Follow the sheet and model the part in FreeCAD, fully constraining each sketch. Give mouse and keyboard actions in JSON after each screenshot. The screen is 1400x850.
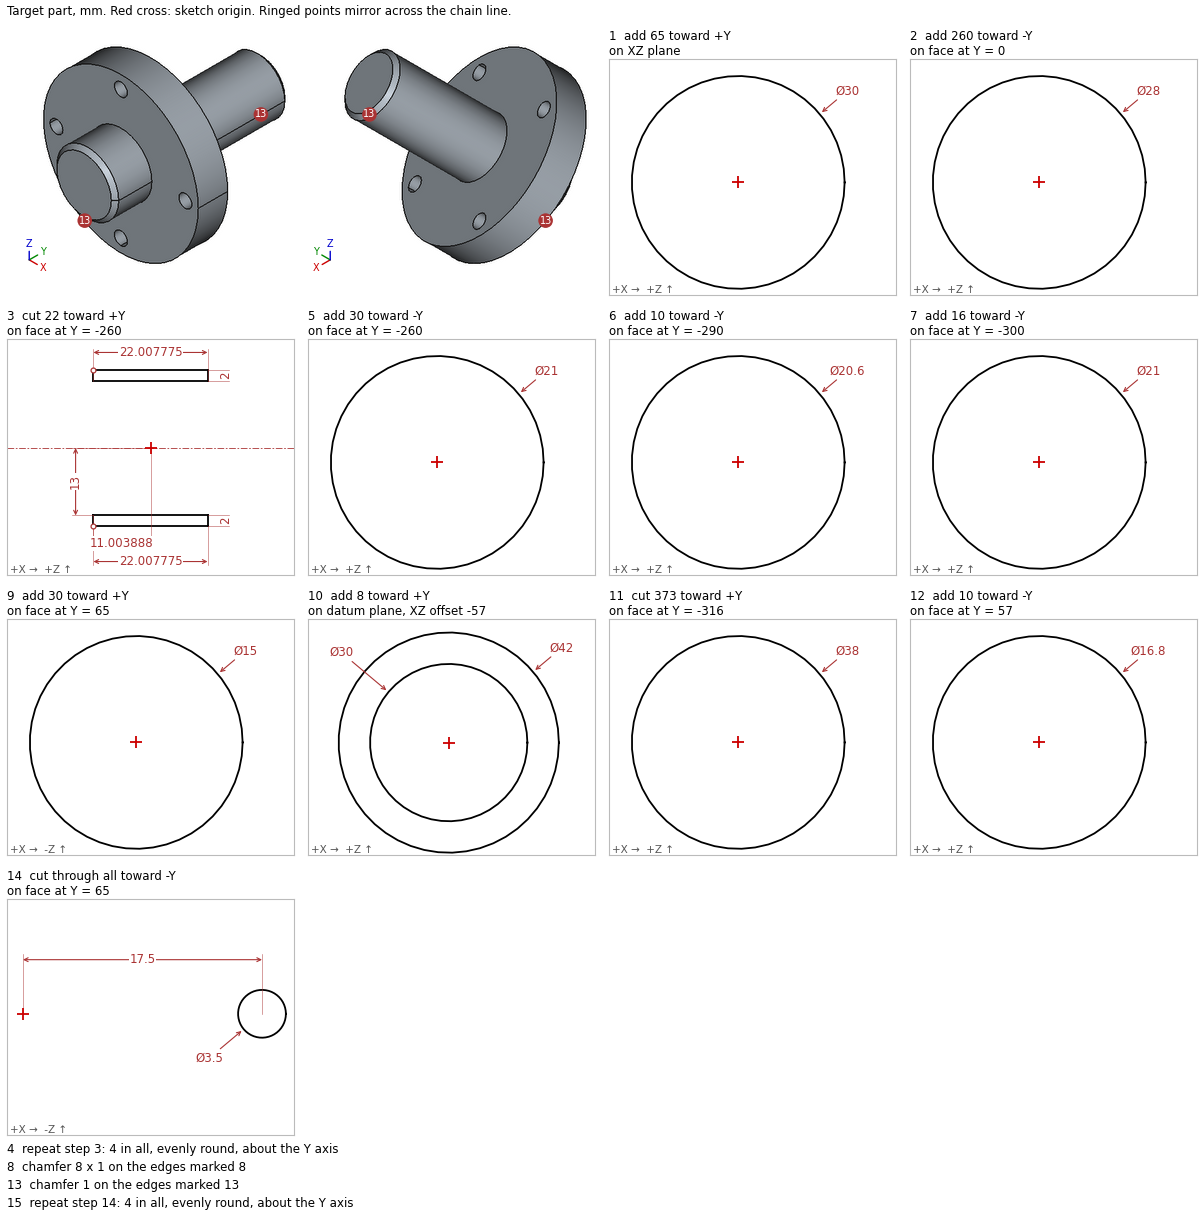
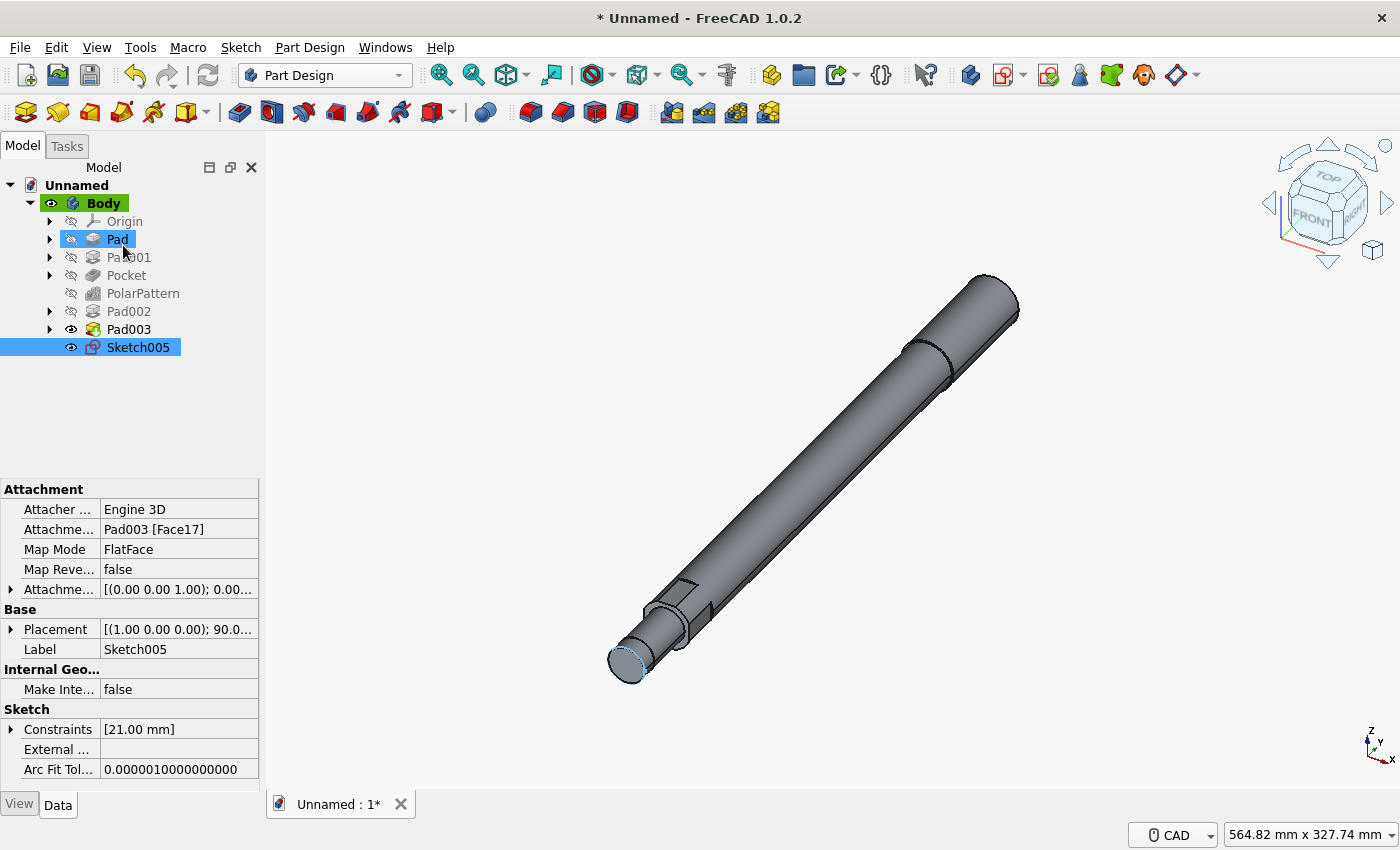
{"action": "left_click", "coordinate": [26, 112]}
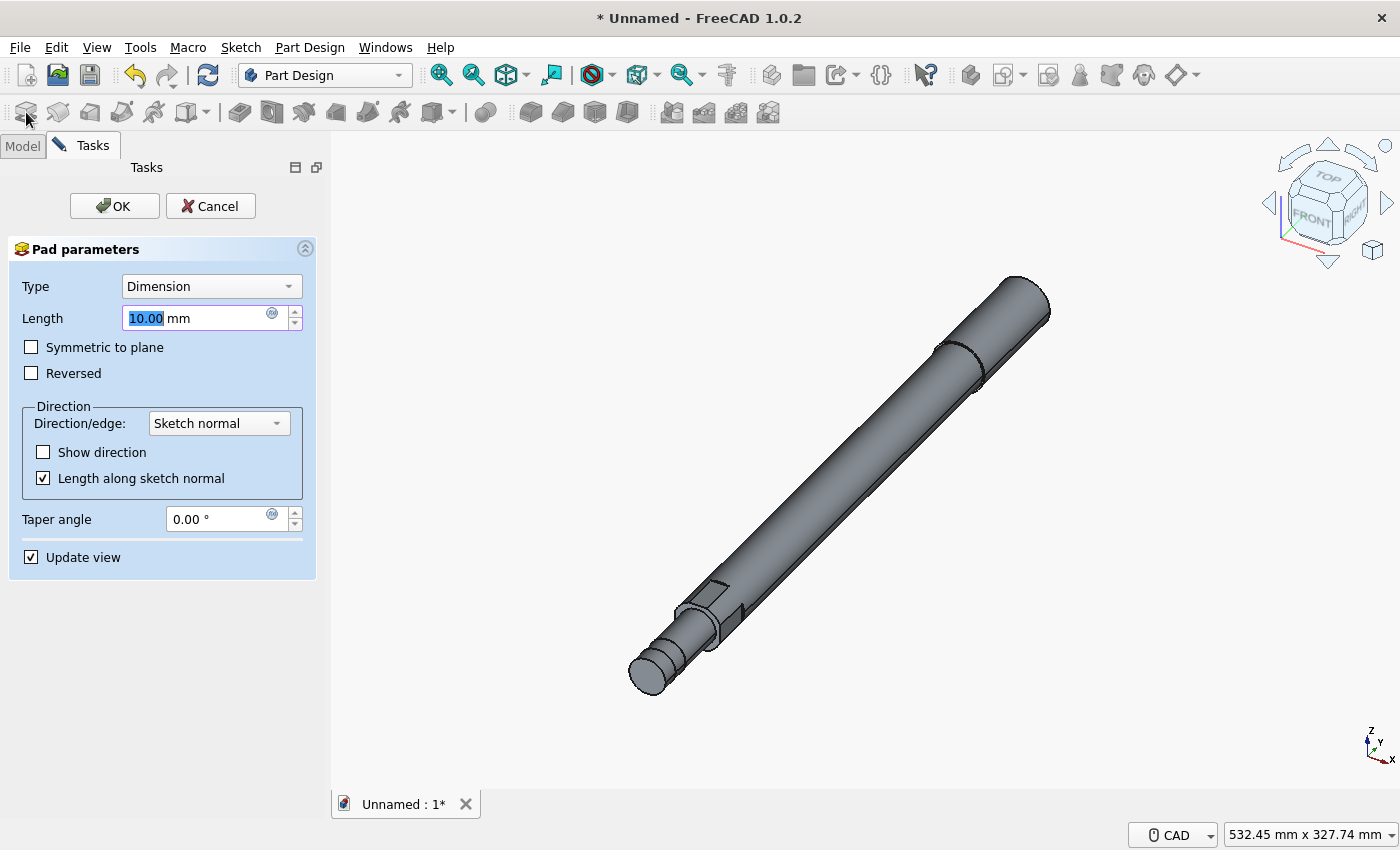
{"action": "type", "text": "16"}
{"action": "key", "text": "Tab"}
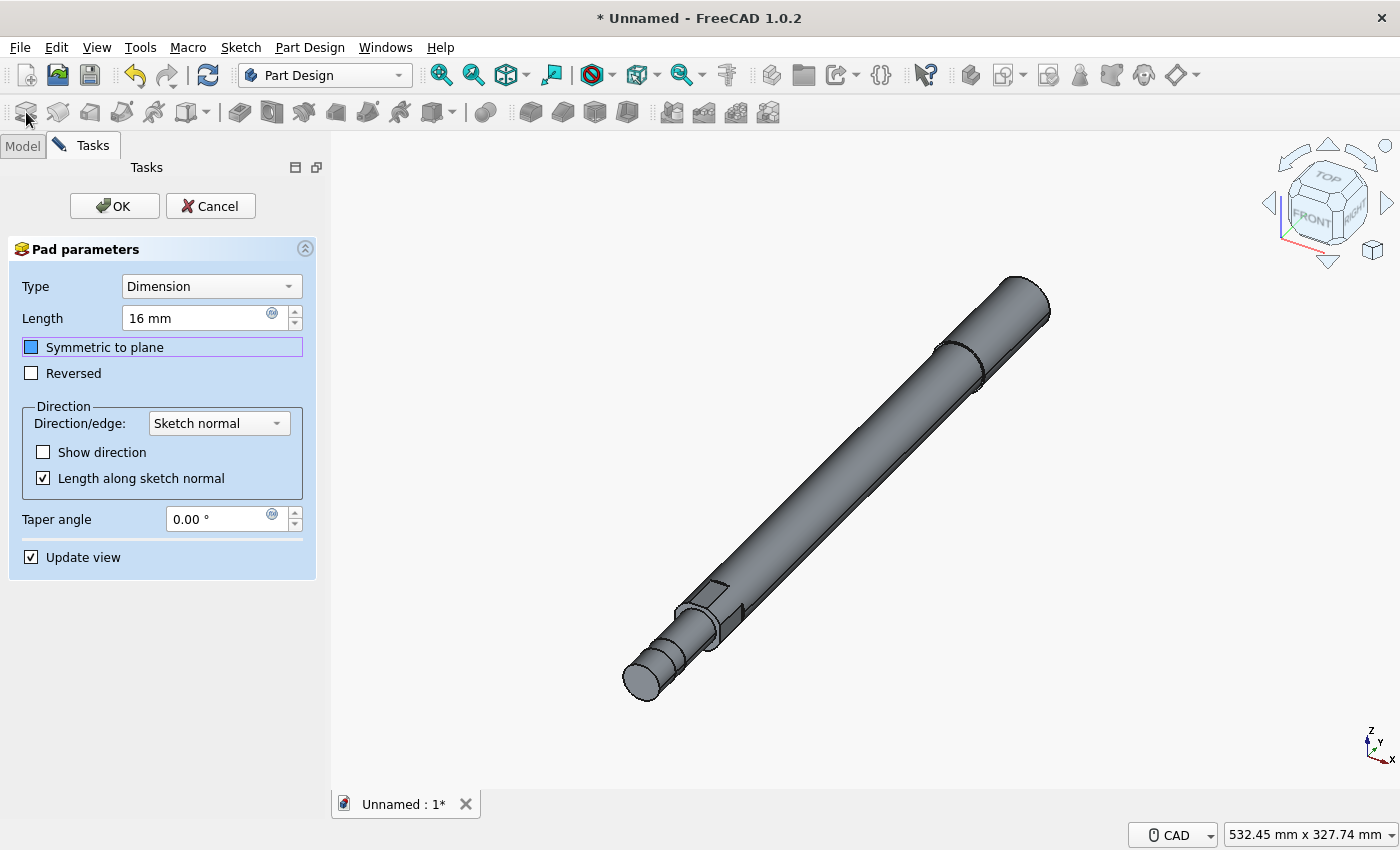
{"action": "left_click", "coordinate": [115, 206]}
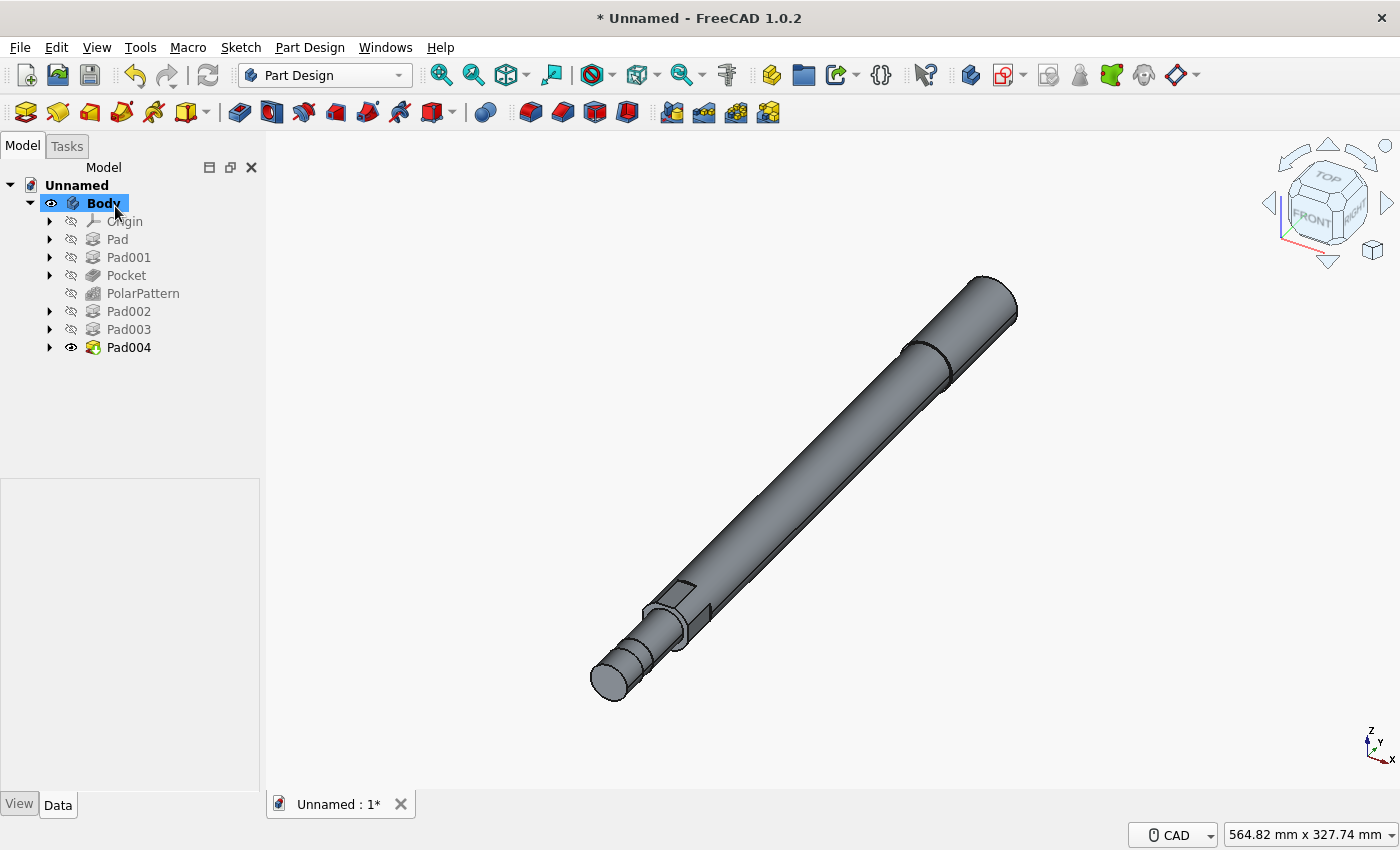
{"action": "left_click", "coordinate": [591, 676]}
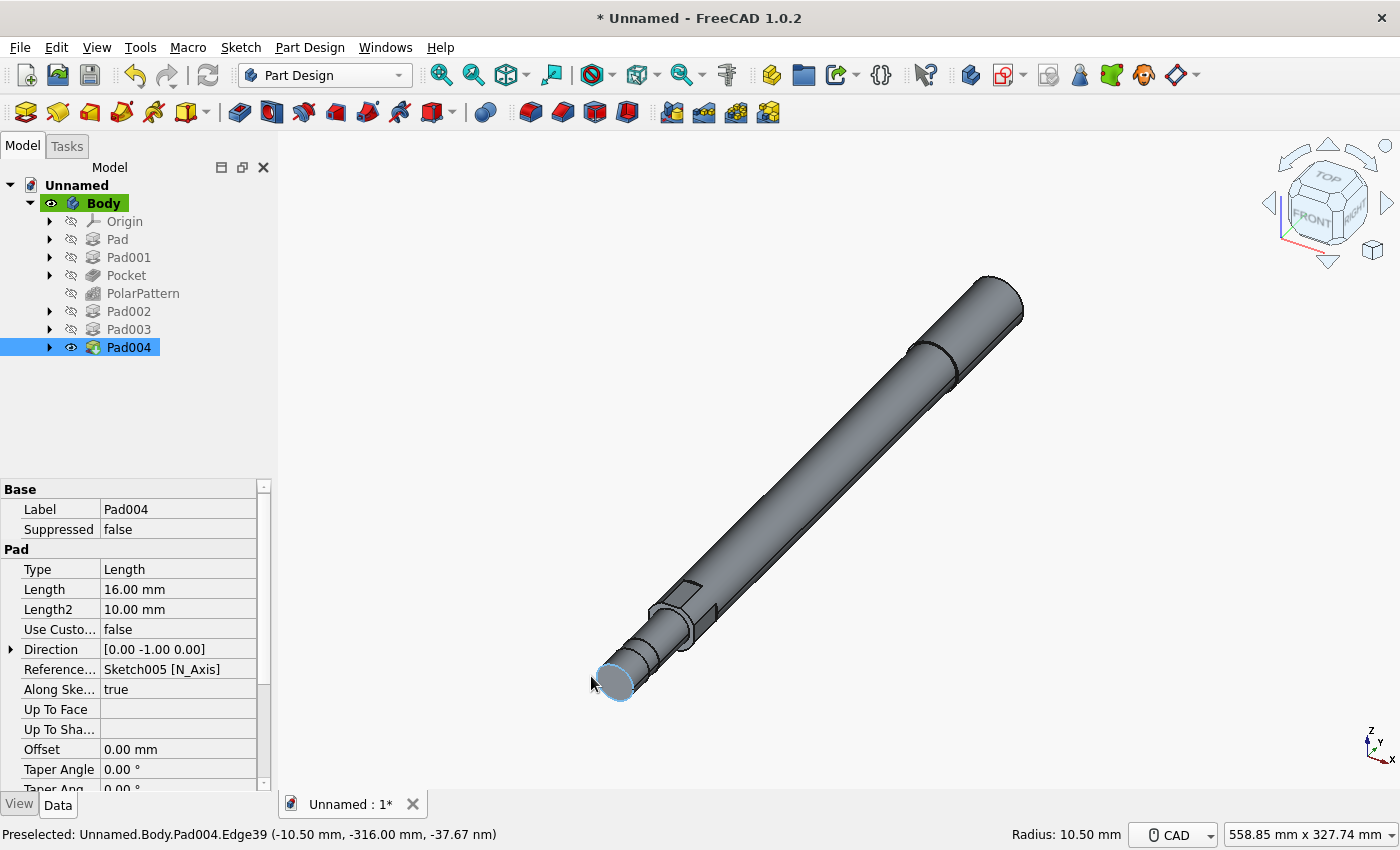
{"action": "left_click", "coordinate": [564, 112]}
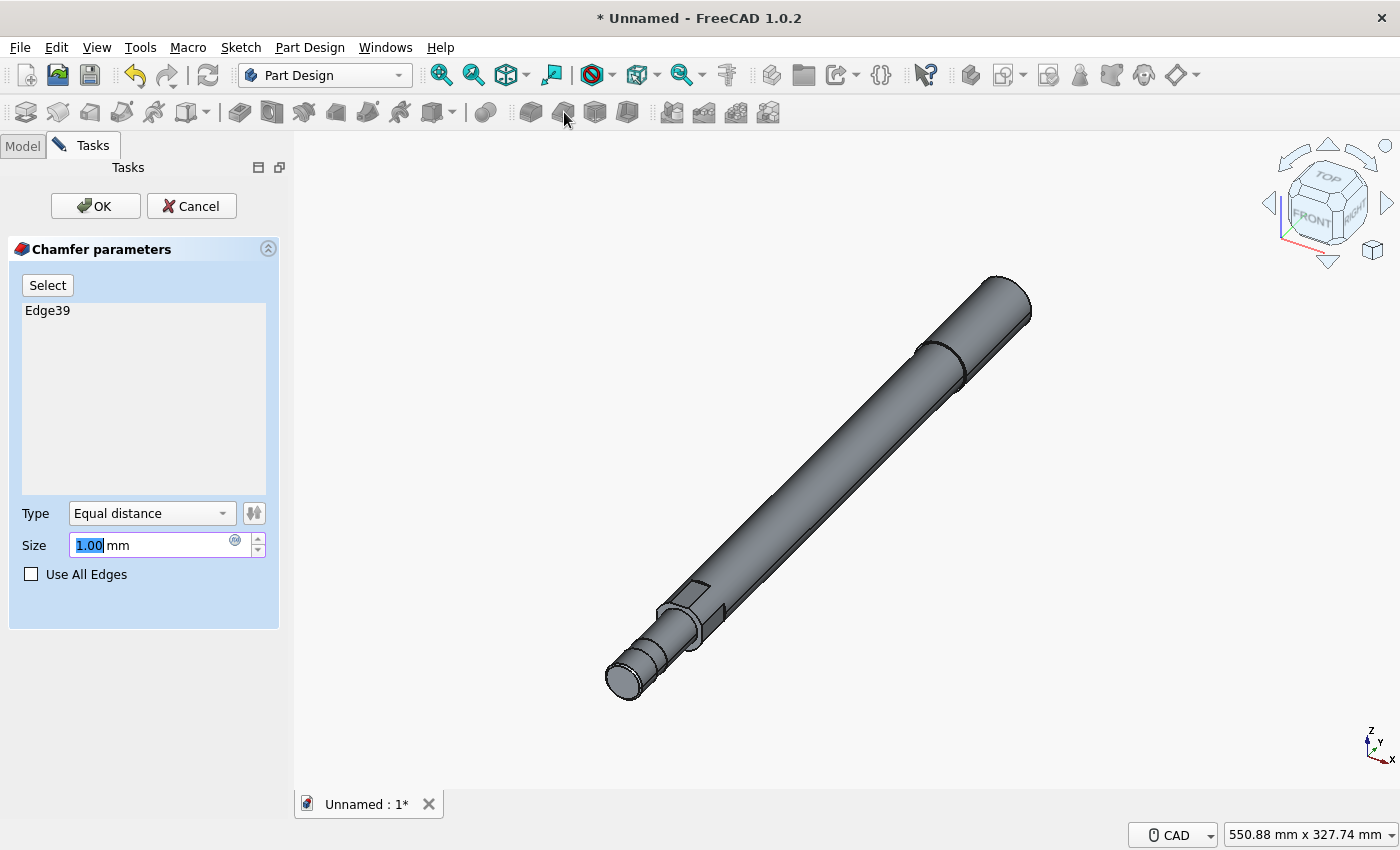
{"action": "type", "text": "8"}
{"action": "key", "text": "Tab"}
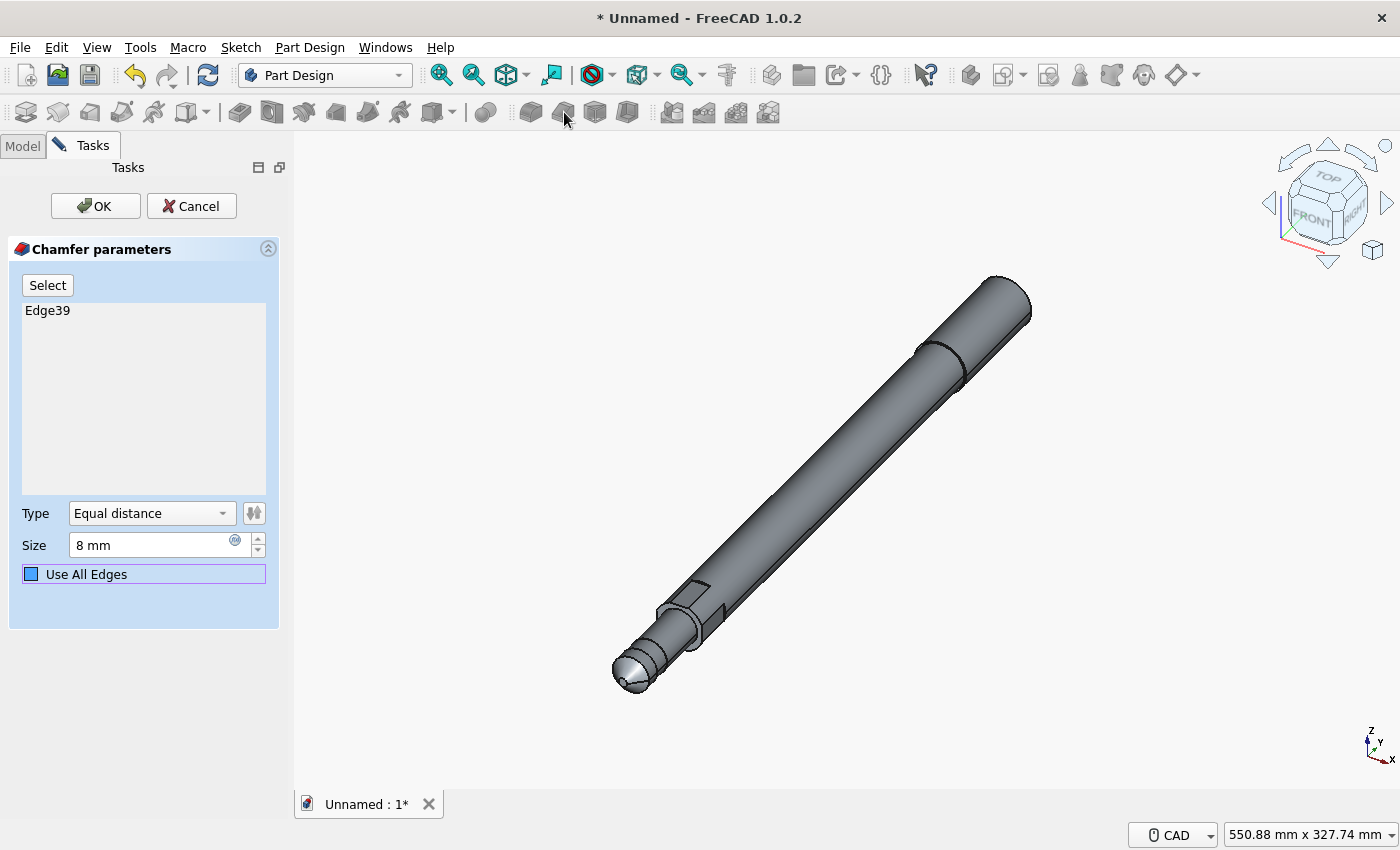
{"action": "left_click", "coordinate": [153, 514]}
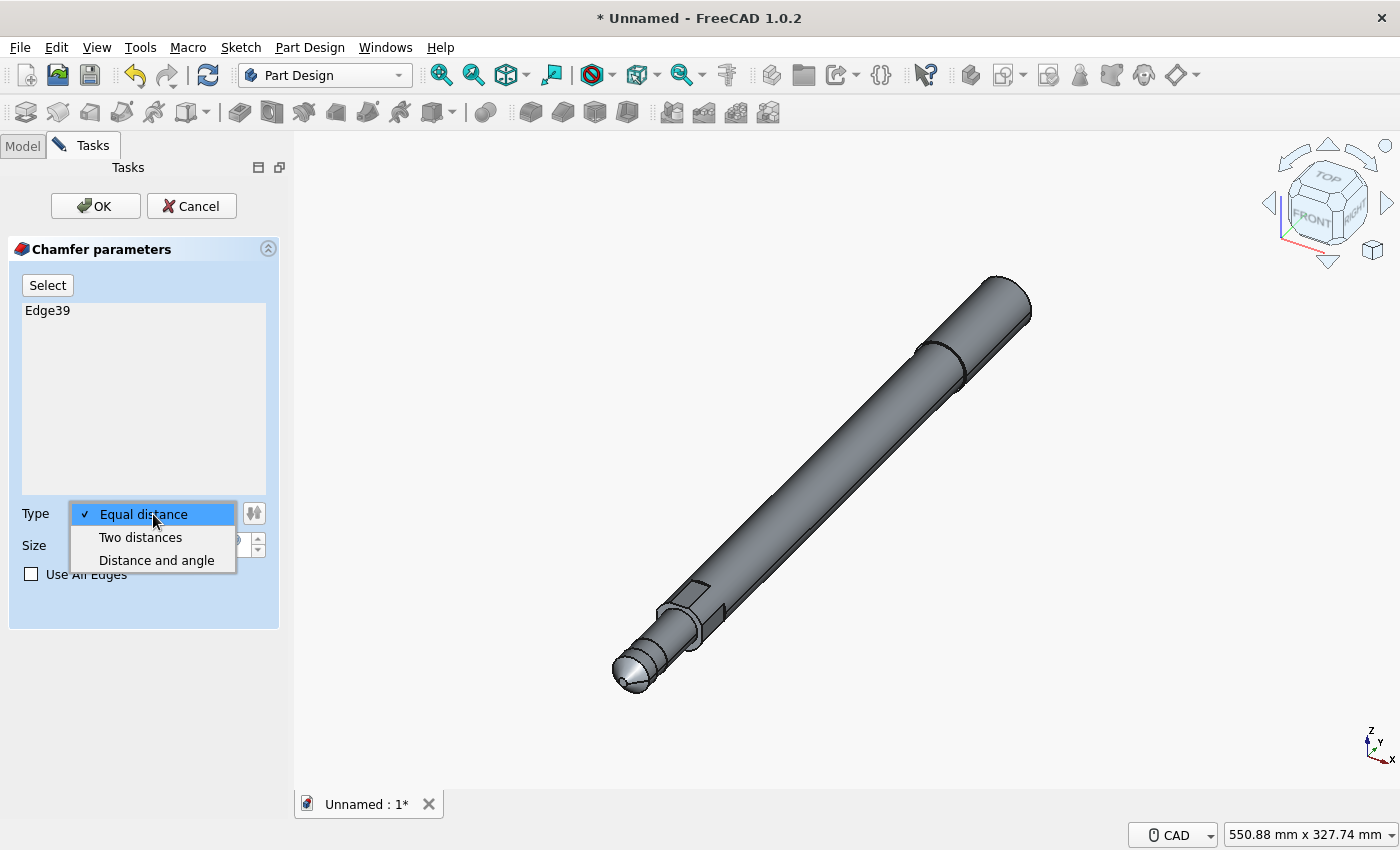
{"action": "left_click", "coordinate": [152, 538]}